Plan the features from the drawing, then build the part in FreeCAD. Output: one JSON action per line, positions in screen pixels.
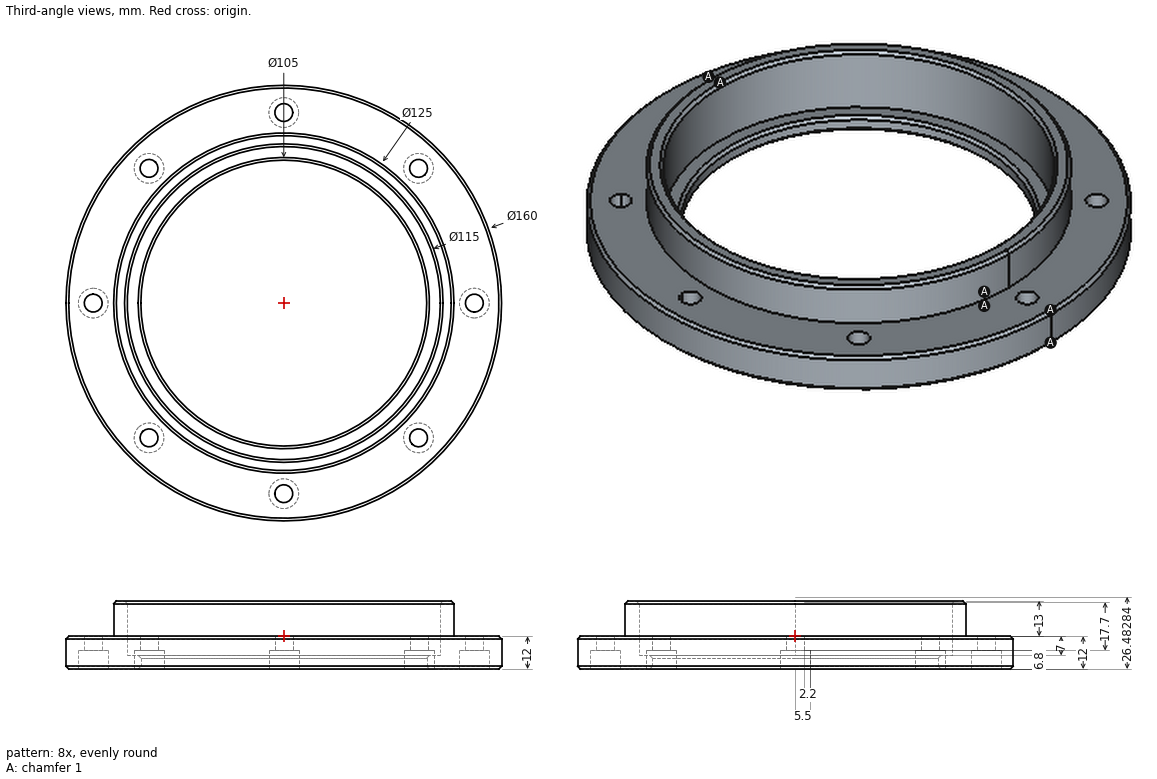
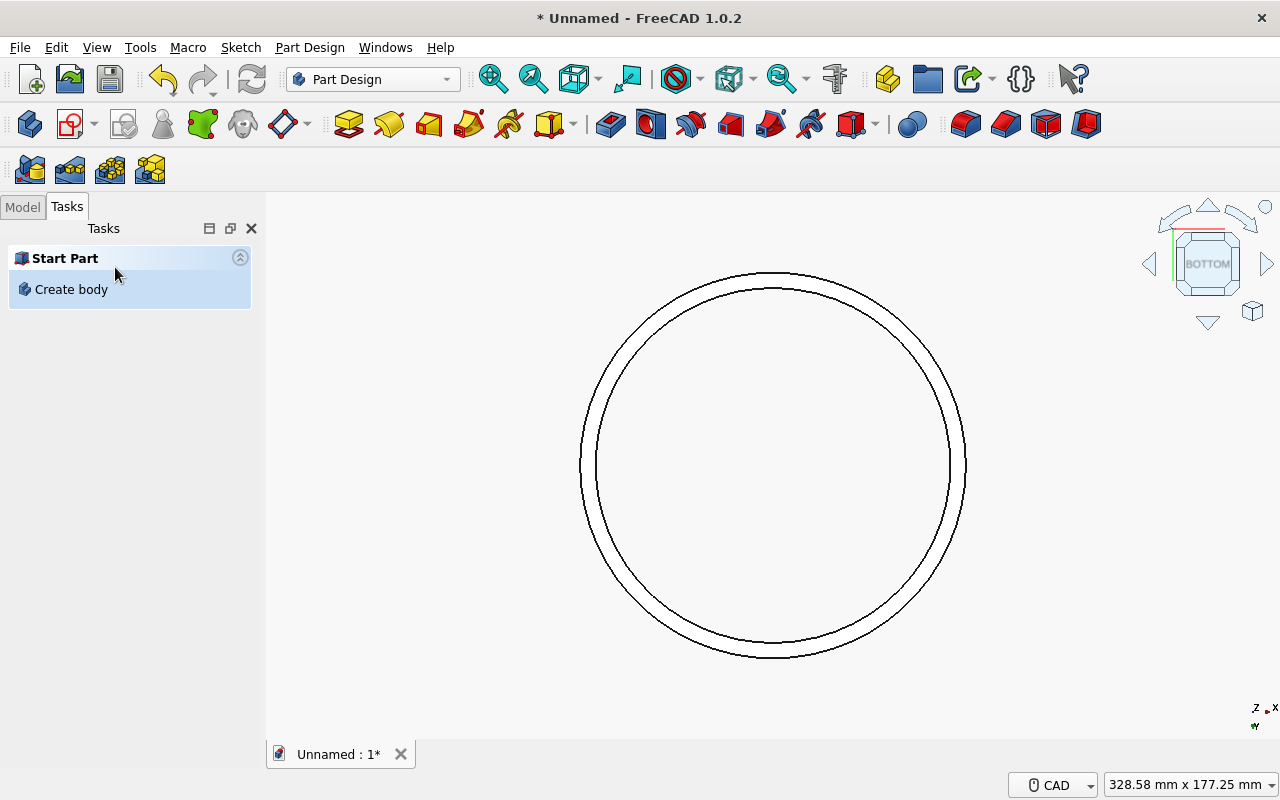
{"action": "left_click", "coordinate": [861, 630]}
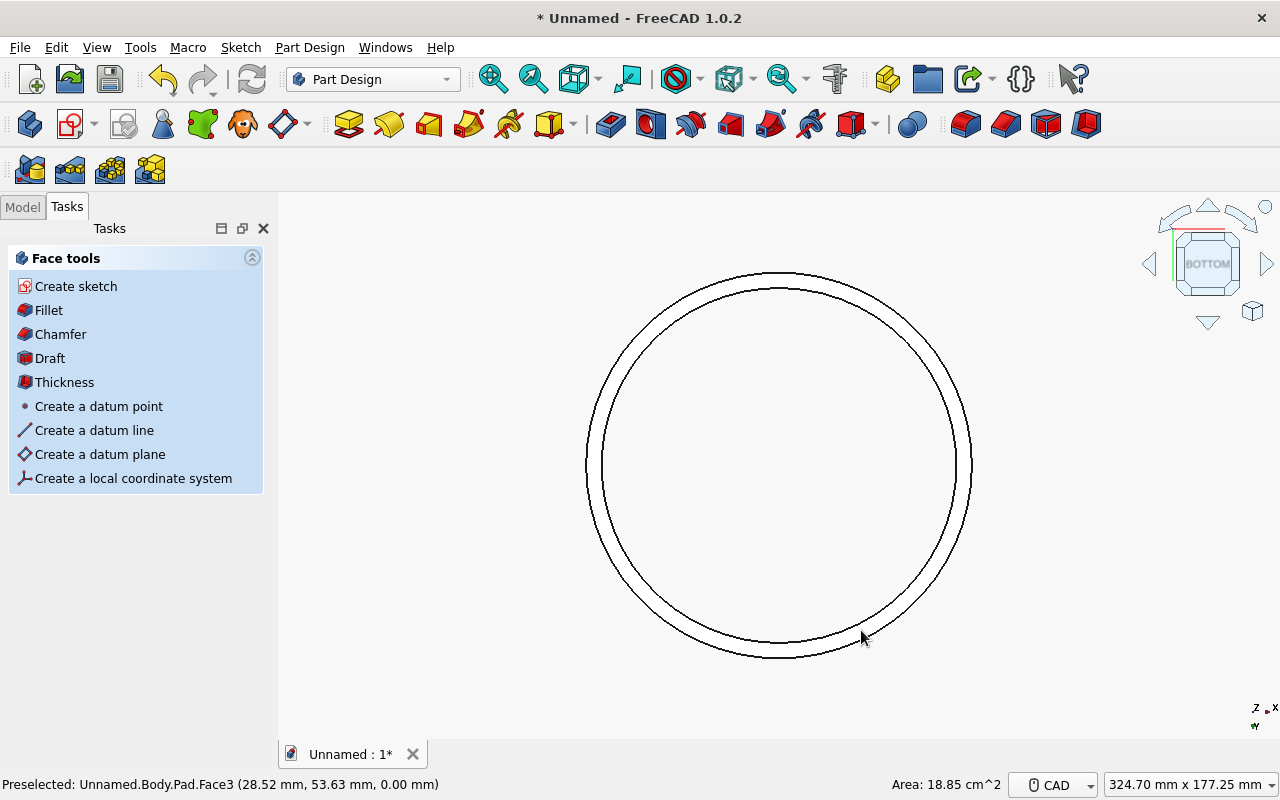
{"action": "left_click", "coordinate": [70, 124]}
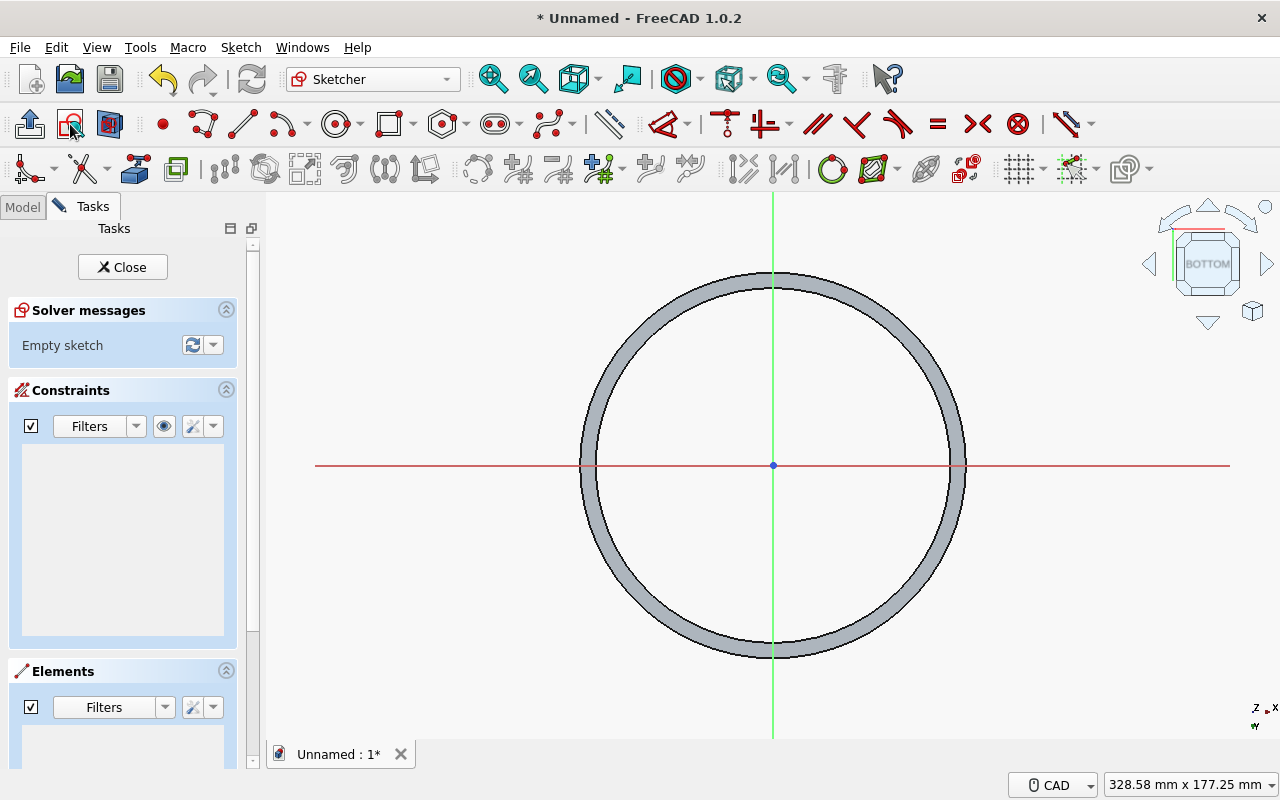
{"action": "scroll", "coordinate": [565, 466], "scroll_direction": "down", "scroll_amount": 2}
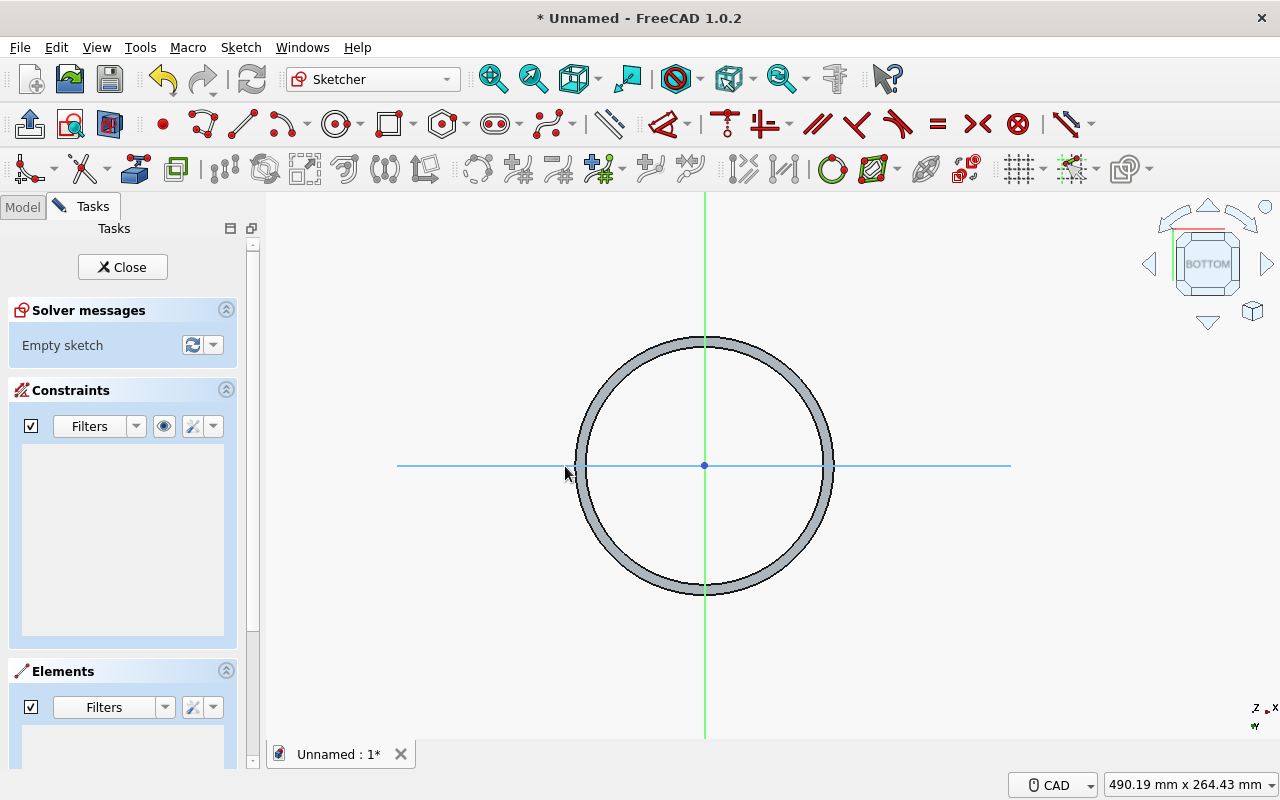
{"action": "key", "text": "g c"}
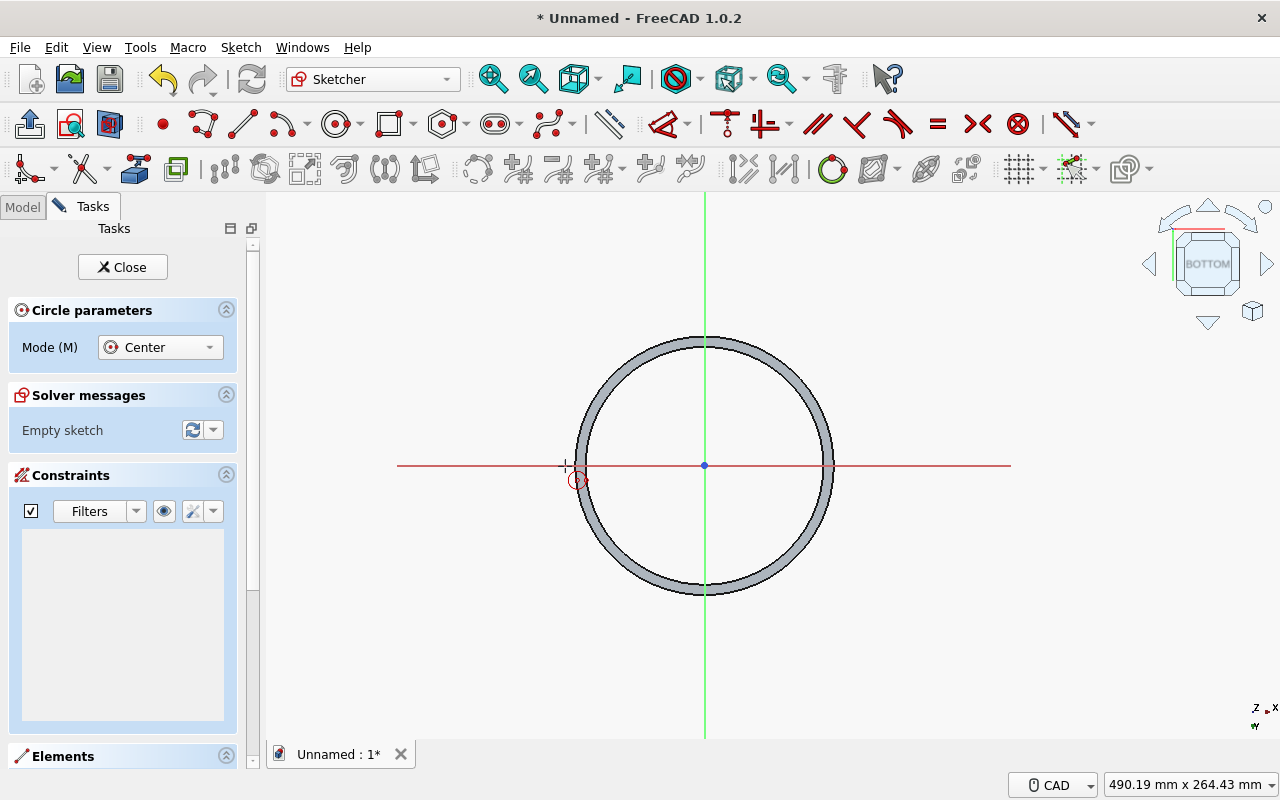
{"action": "left_click", "coordinate": [705, 466]}
{"action": "left_click", "coordinate": [822, 349]}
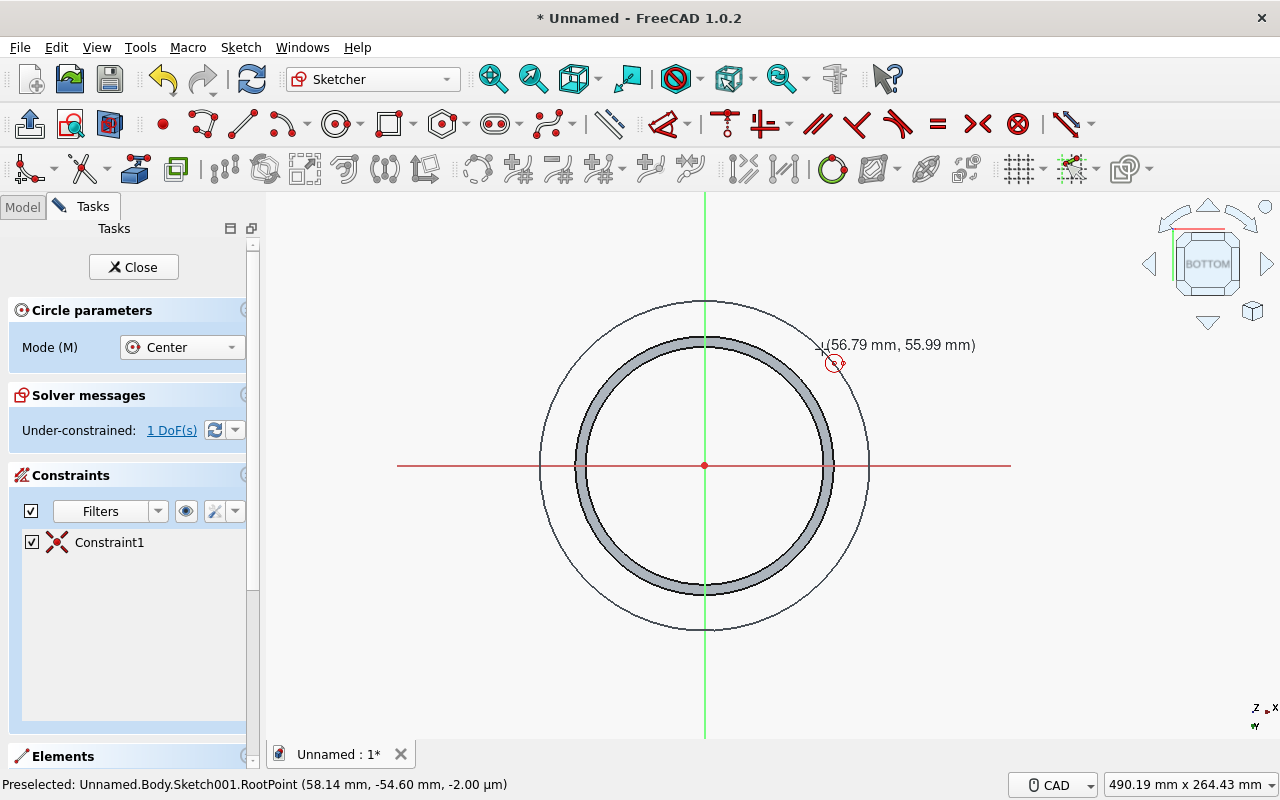
{"action": "left_click", "coordinate": [705, 466]}
{"action": "left_click", "coordinate": [781, 389]}
{"action": "key", "text": "Escape"}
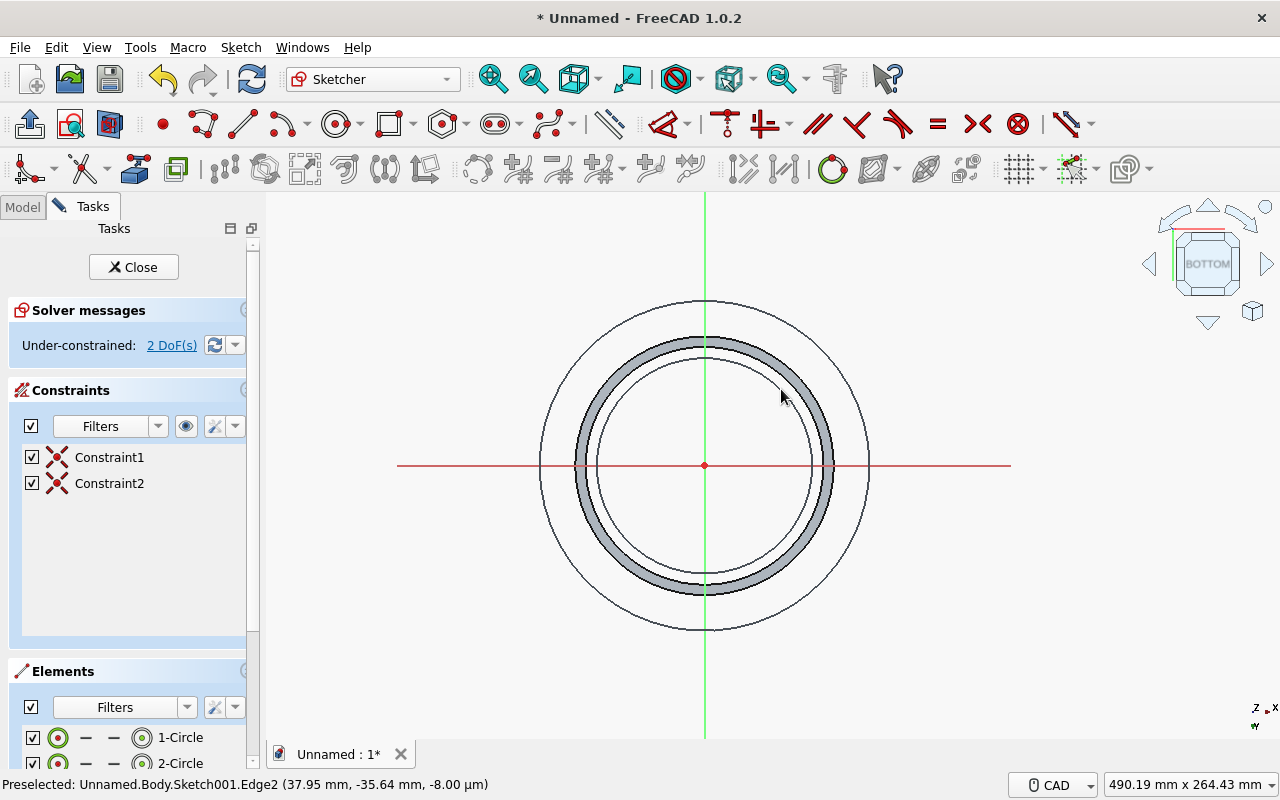
{"action": "left_click", "coordinate": [821, 349]}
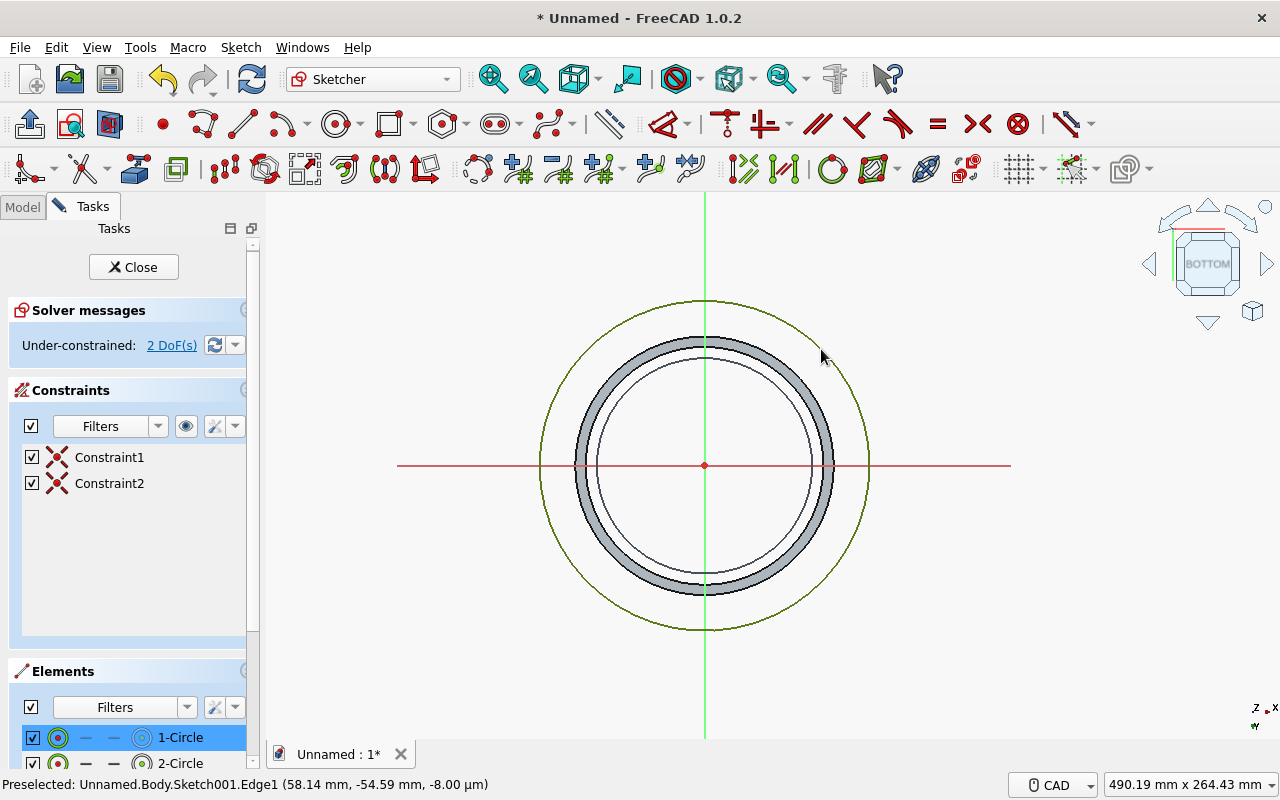
{"action": "key", "text": "k o"}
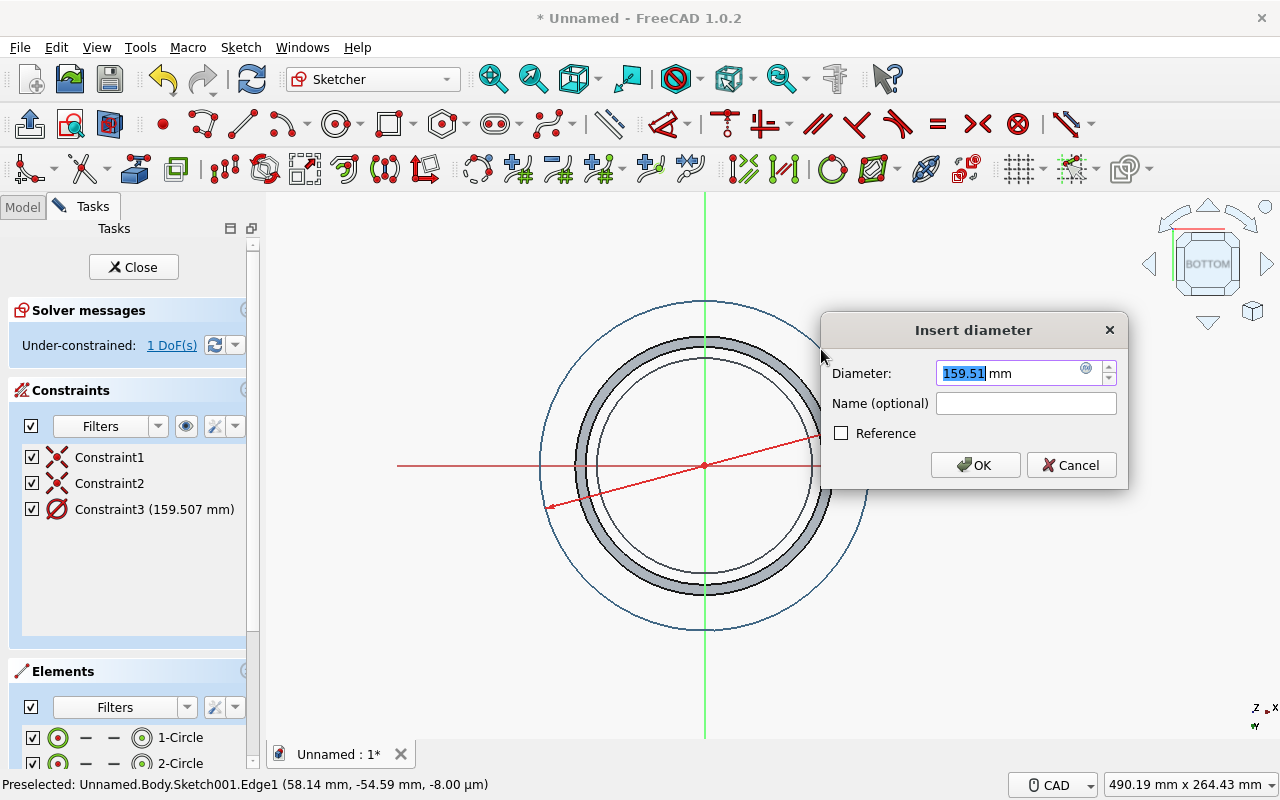
{"action": "type", "text": "160"}
{"action": "key", "text": "Return"}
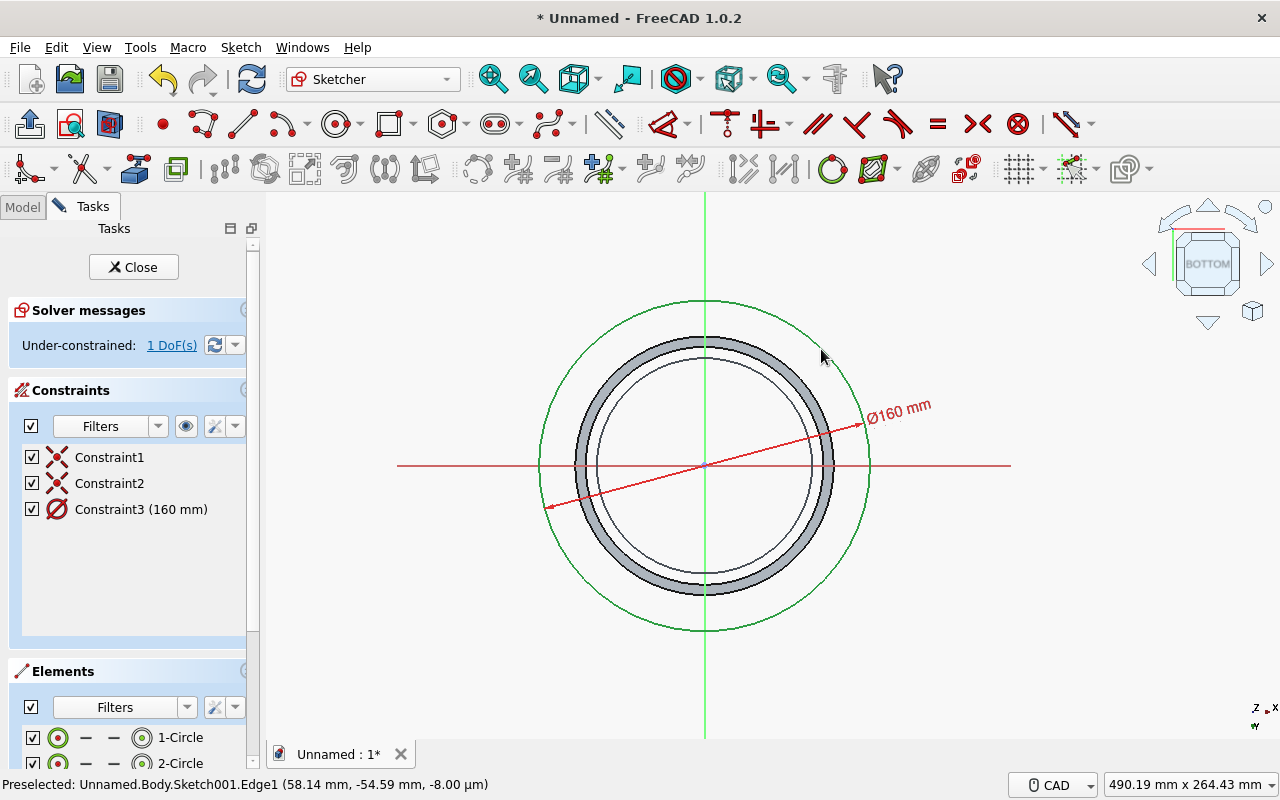
{"action": "left_click", "coordinate": [780, 389]}